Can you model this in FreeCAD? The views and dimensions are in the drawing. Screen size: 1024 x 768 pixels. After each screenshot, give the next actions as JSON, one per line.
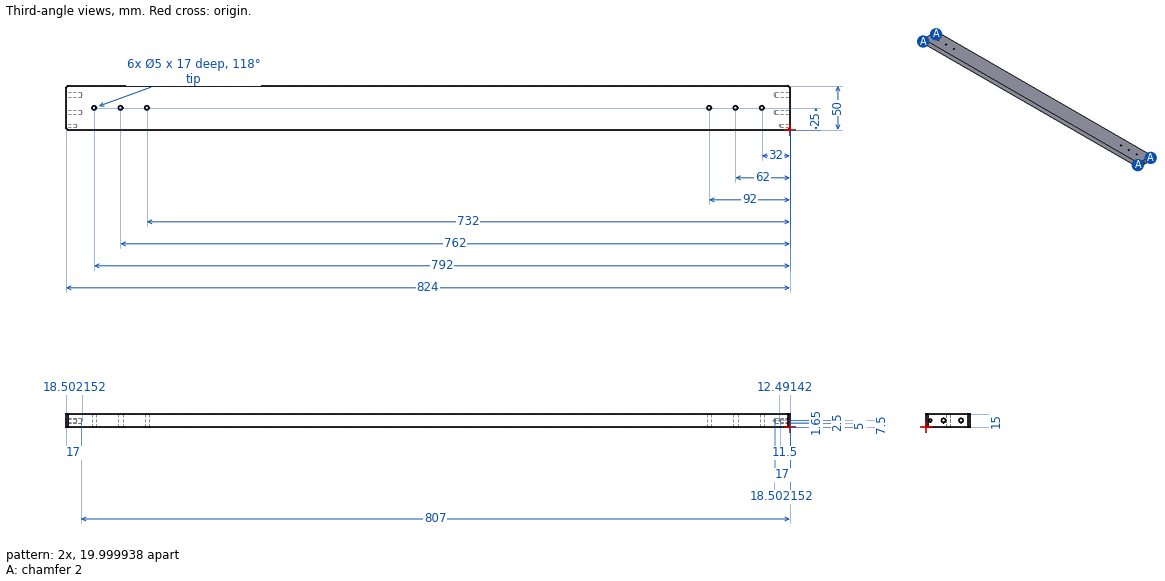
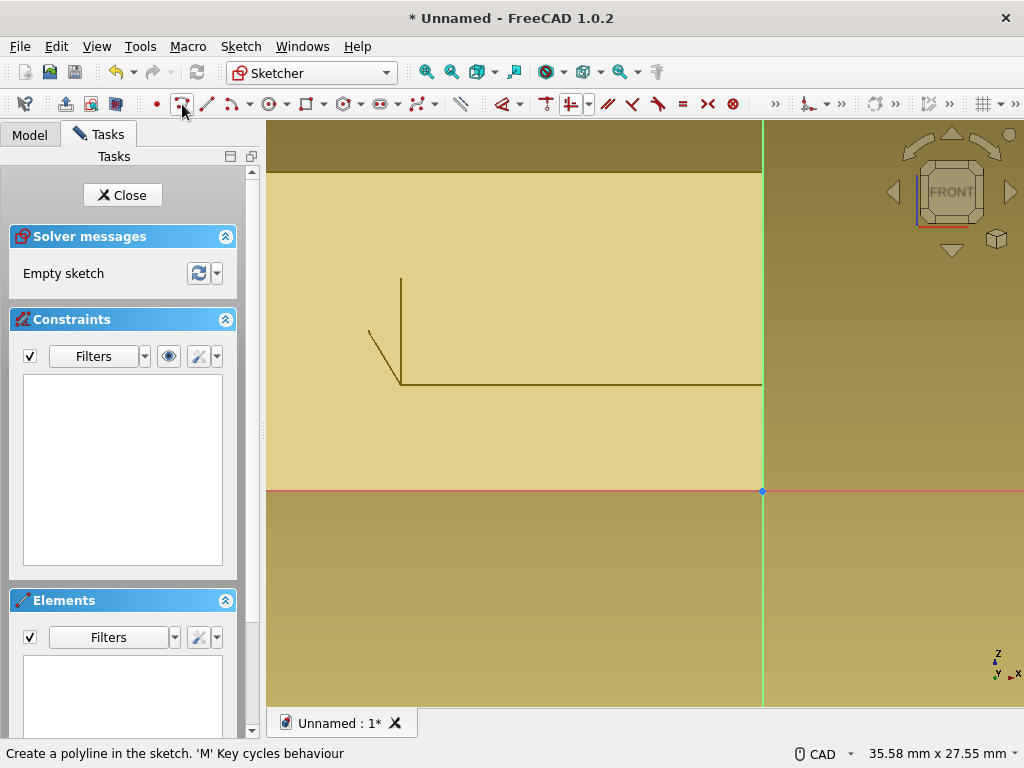
{"action": "left_click", "coordinate": [763, 367]}
{"action": "left_click", "coordinate": [518, 367]}
{"action": "left_click", "coordinate": [497, 331]}
{"action": "left_click", "coordinate": [754, 331]}
{"action": "left_click", "coordinate": [763, 368]}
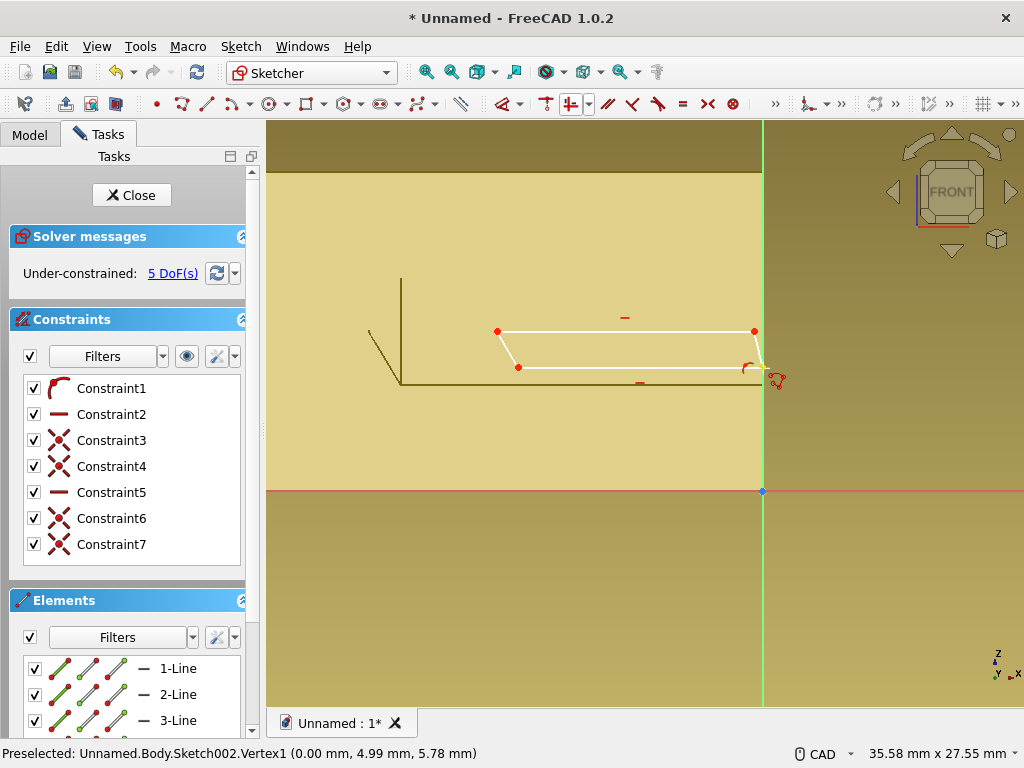
{"action": "left_click", "coordinate": [207, 104]}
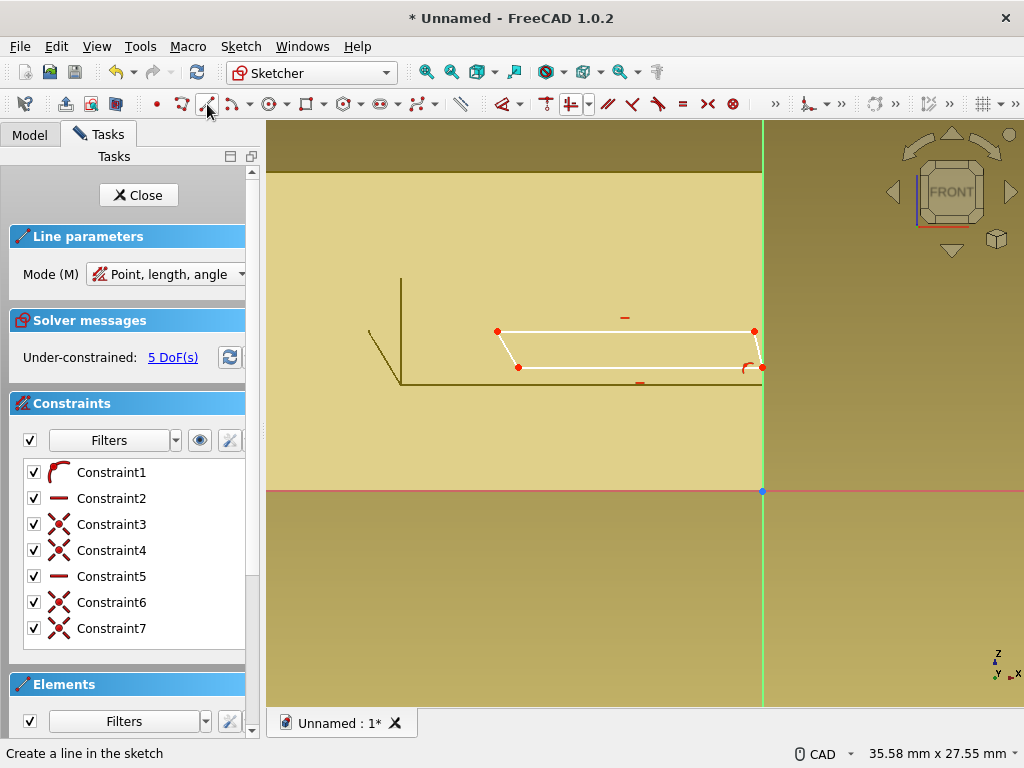
{"action": "left_click", "coordinate": [470, 331]}
{"action": "left_click", "coordinate": [390, 331]}
{"action": "key", "text": "Escape"}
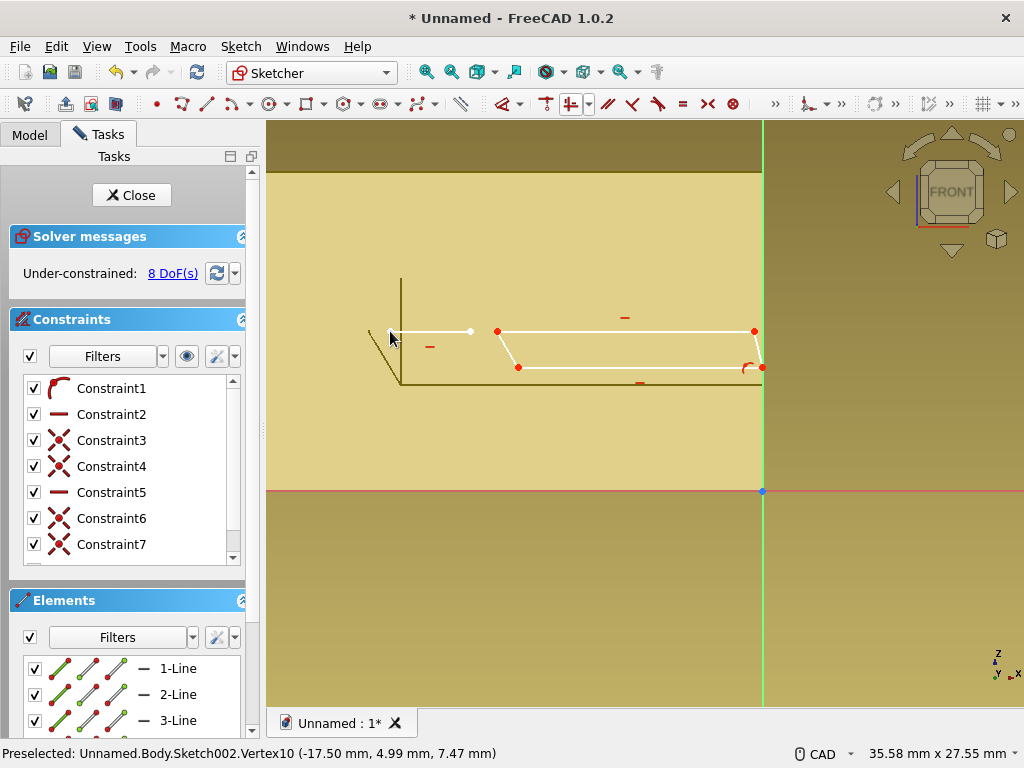
{"action": "left_click", "coordinate": [446, 332]}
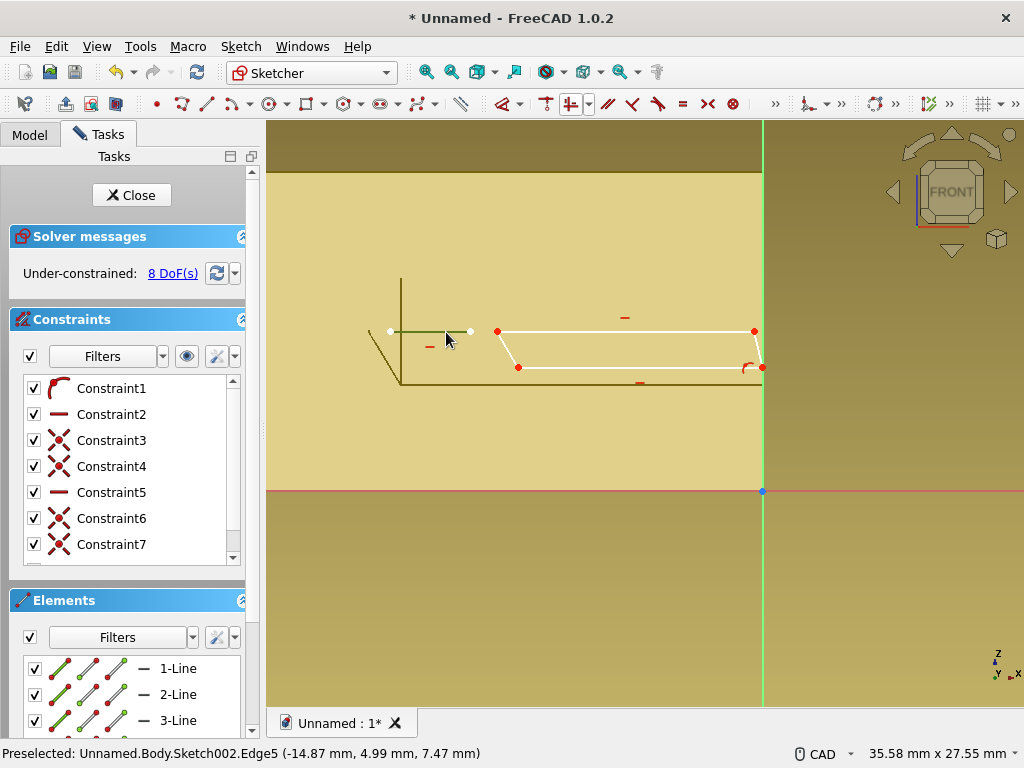
{"action": "left_click", "coordinate": [461, 104]}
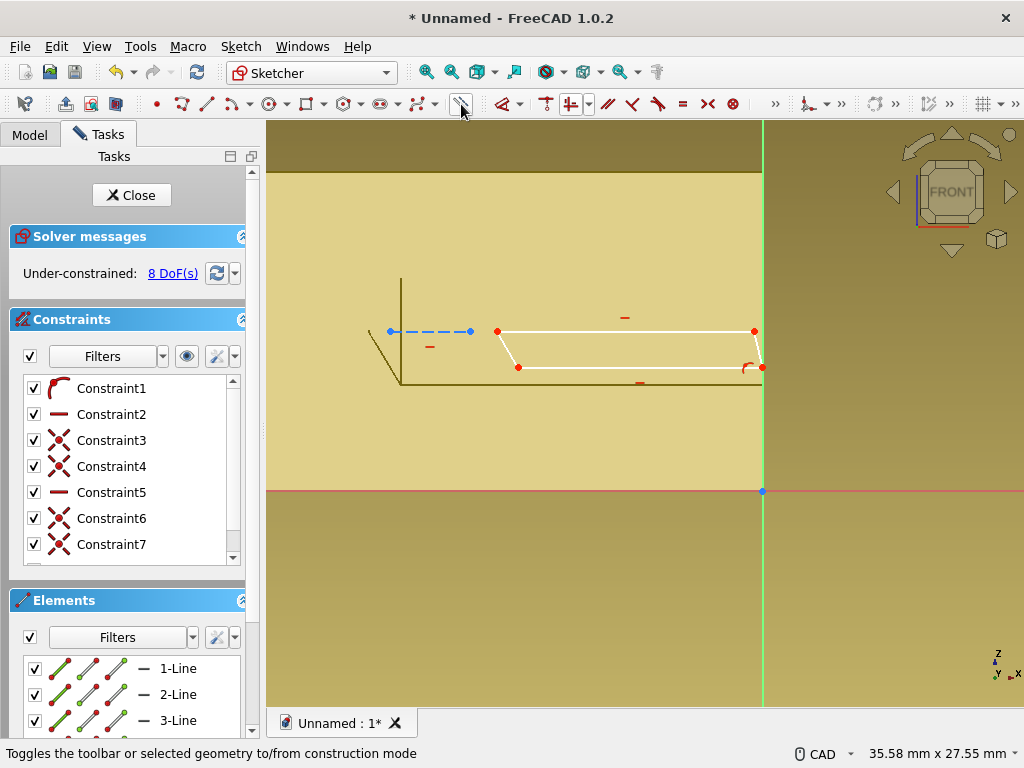
{"action": "scroll", "coordinate": [760, 357], "scroll_direction": "up", "scroll_amount": 2}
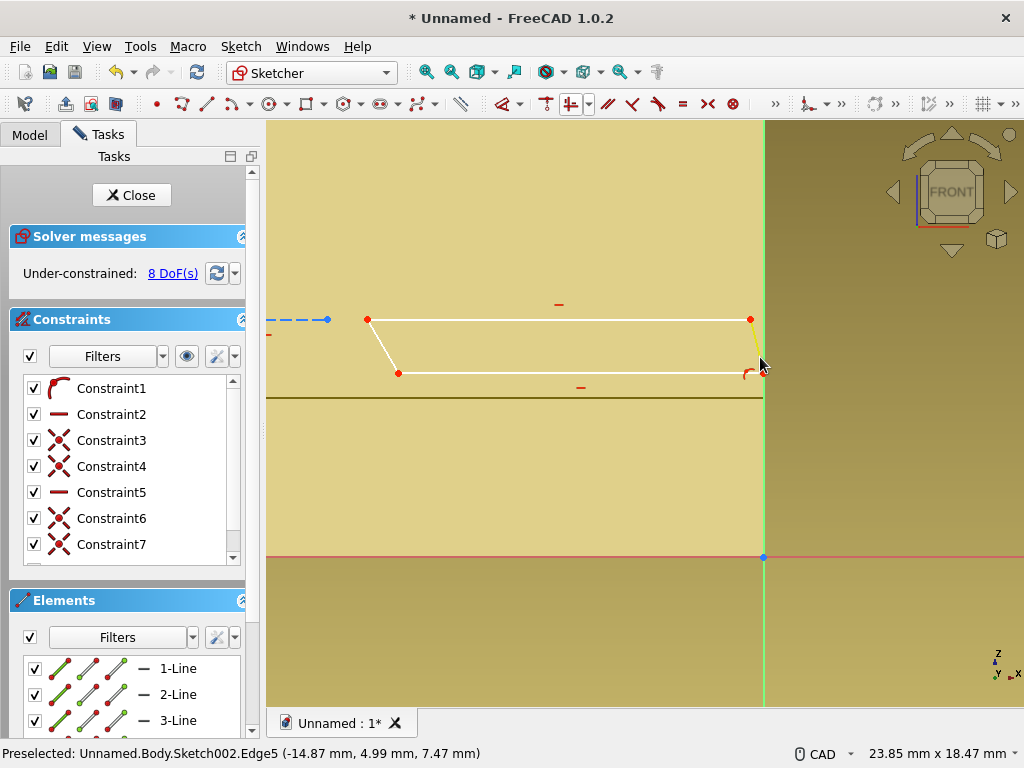
{"action": "left_click", "coordinate": [760, 357]}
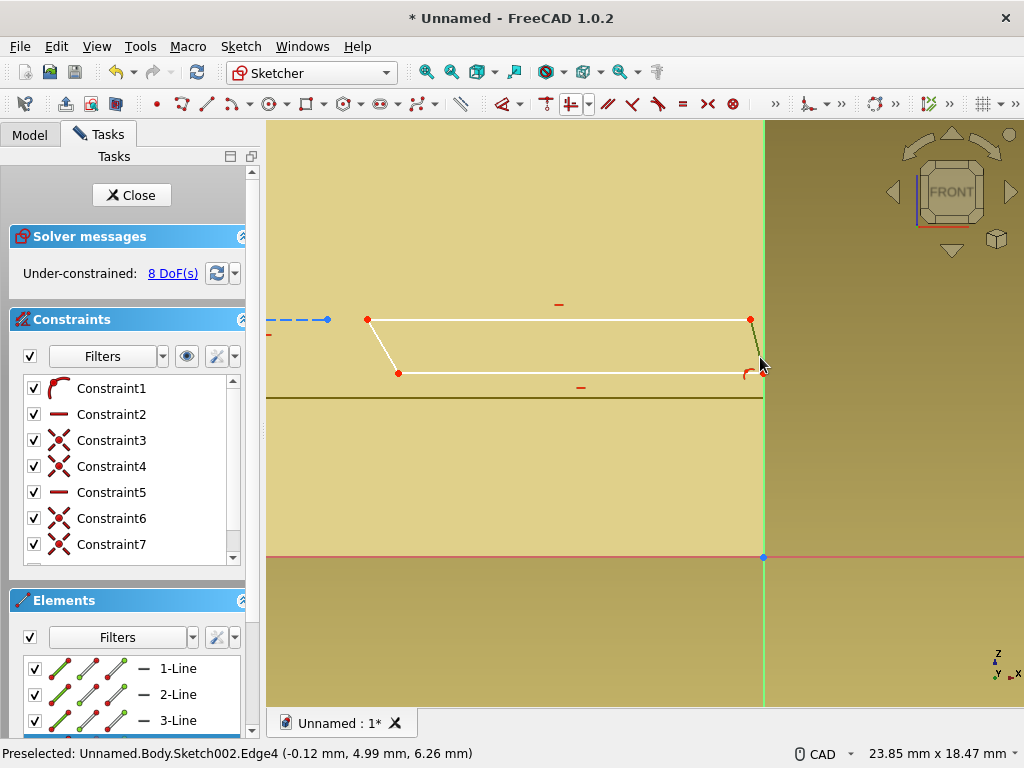
{"action": "left_click", "coordinate": [588, 104]}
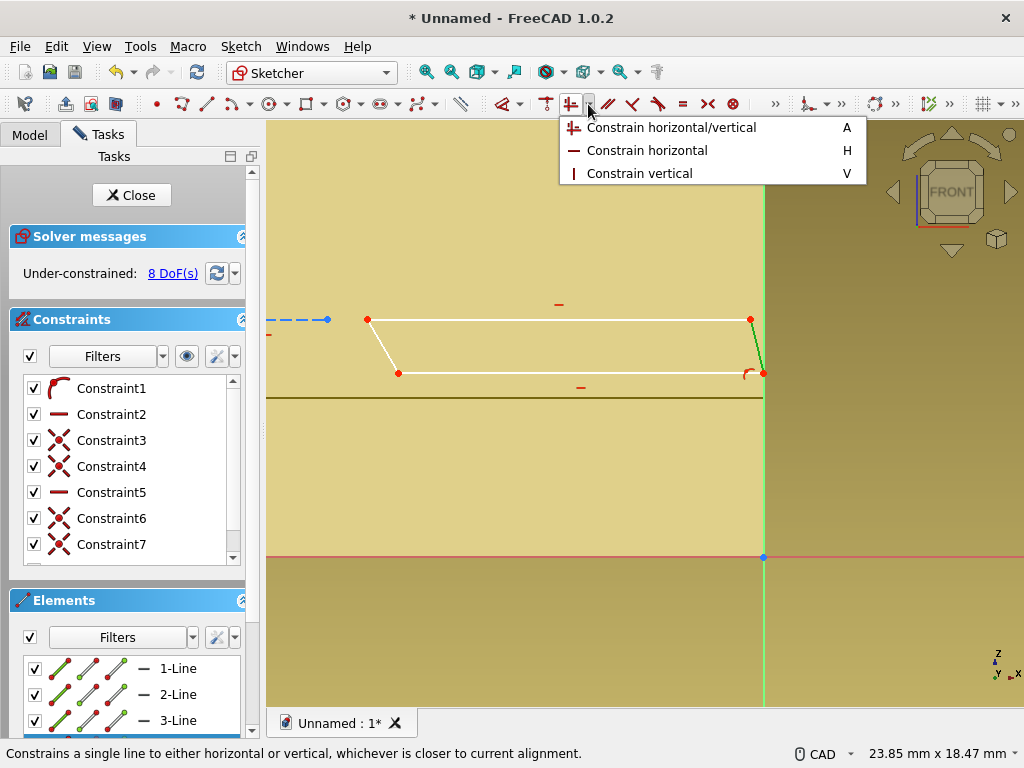
{"action": "left_click", "coordinate": [713, 174]}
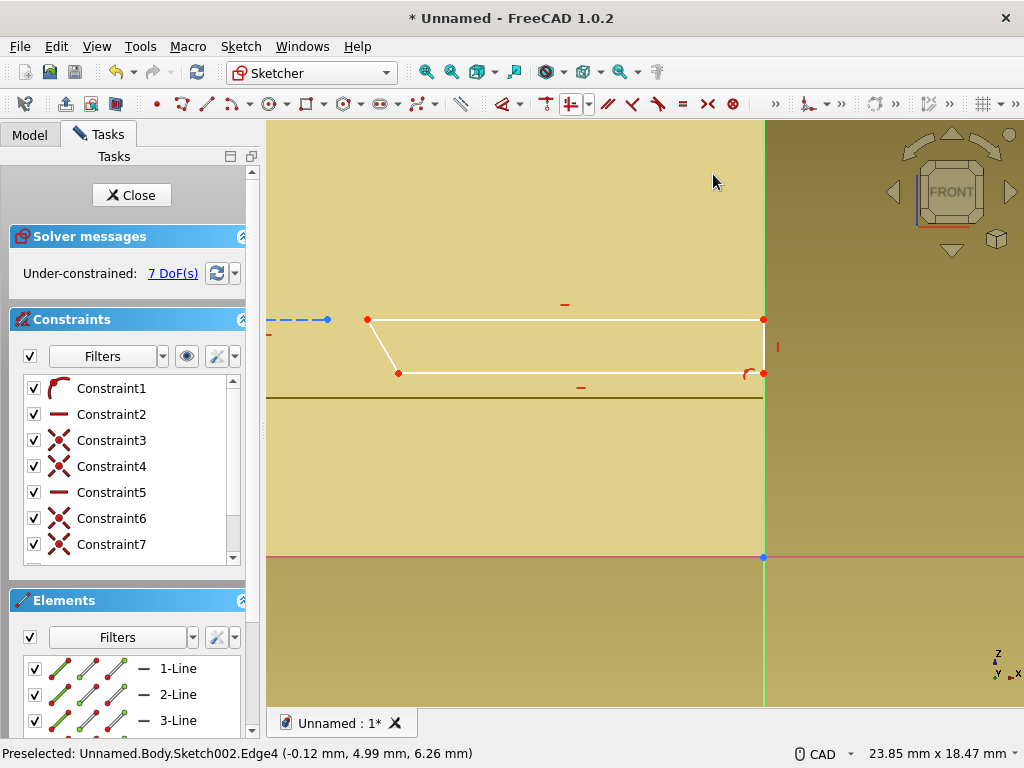
{"action": "left_click", "coordinate": [502, 104]}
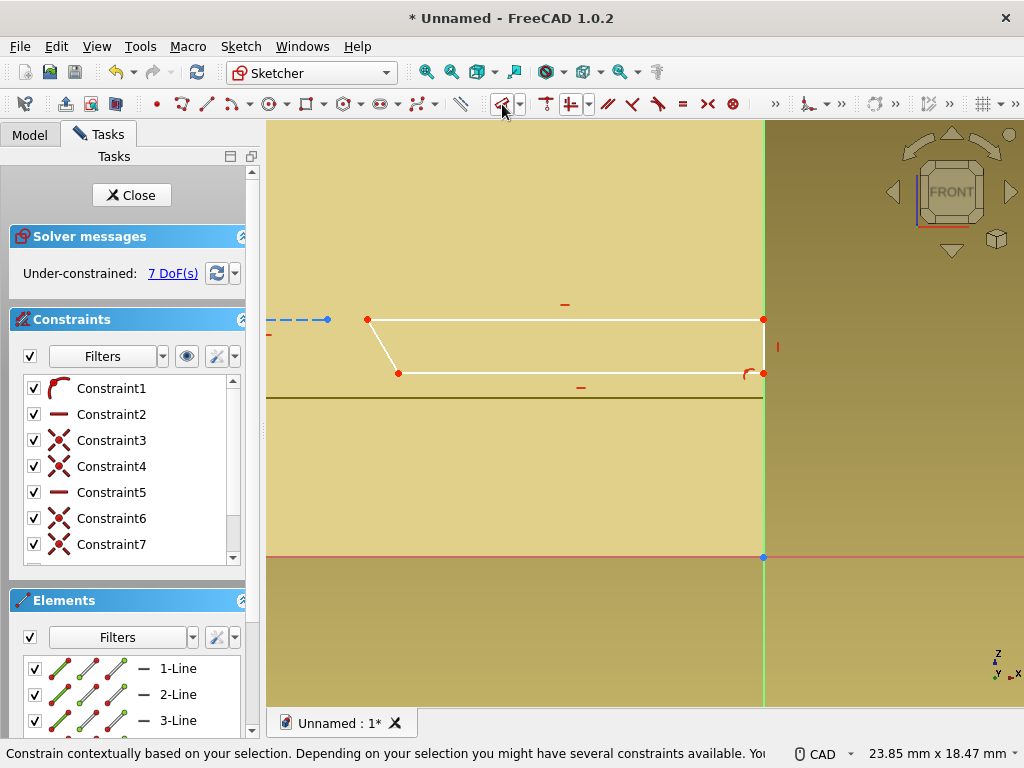
{"action": "left_click", "coordinate": [654, 373]}
{"action": "left_click", "coordinate": [581, 339]}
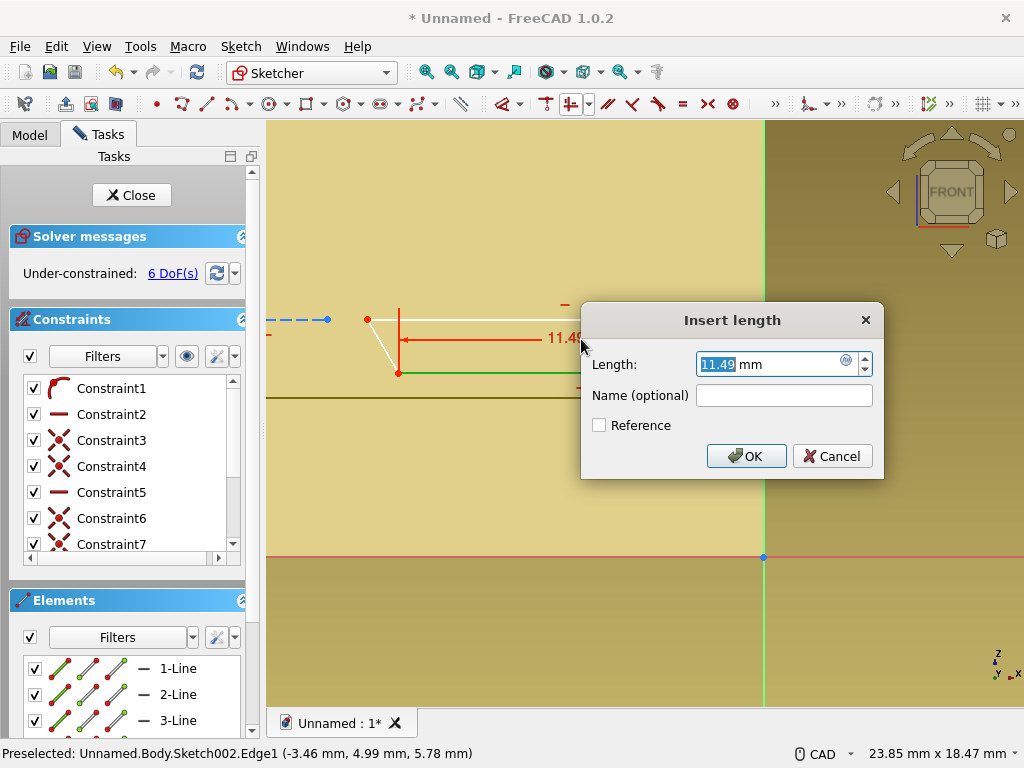
{"action": "type", "text": "11.5"}
{"action": "key", "text": "Return"}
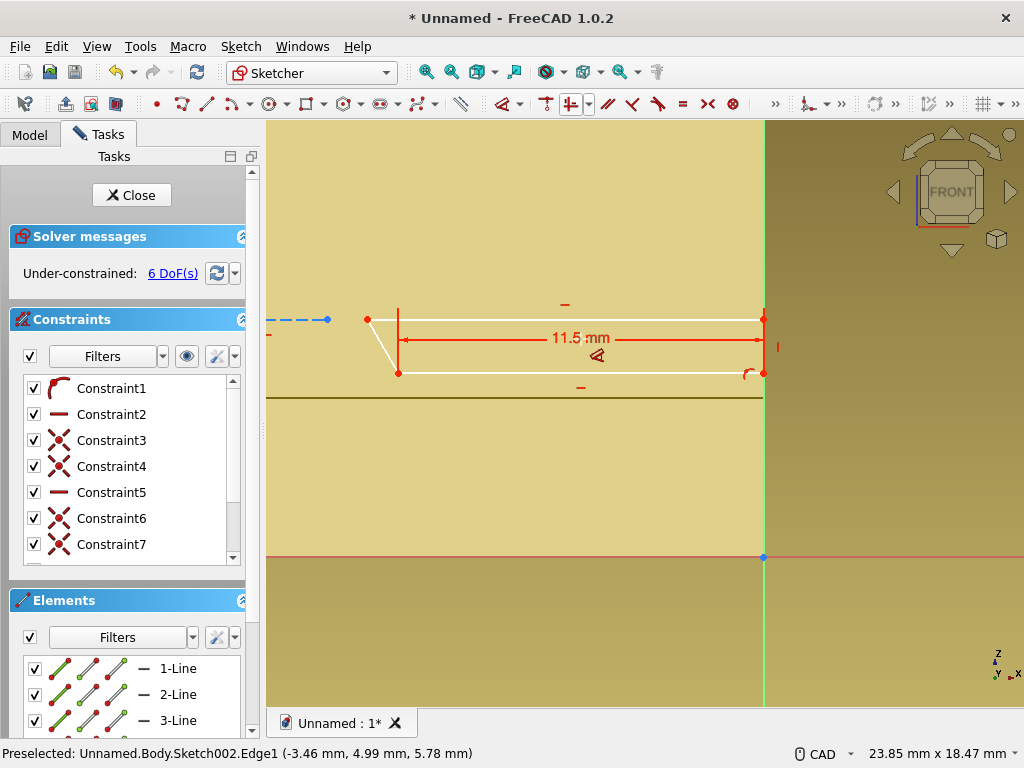
{"action": "left_click", "coordinate": [764, 336]}
{"action": "left_click", "coordinate": [798, 346]}